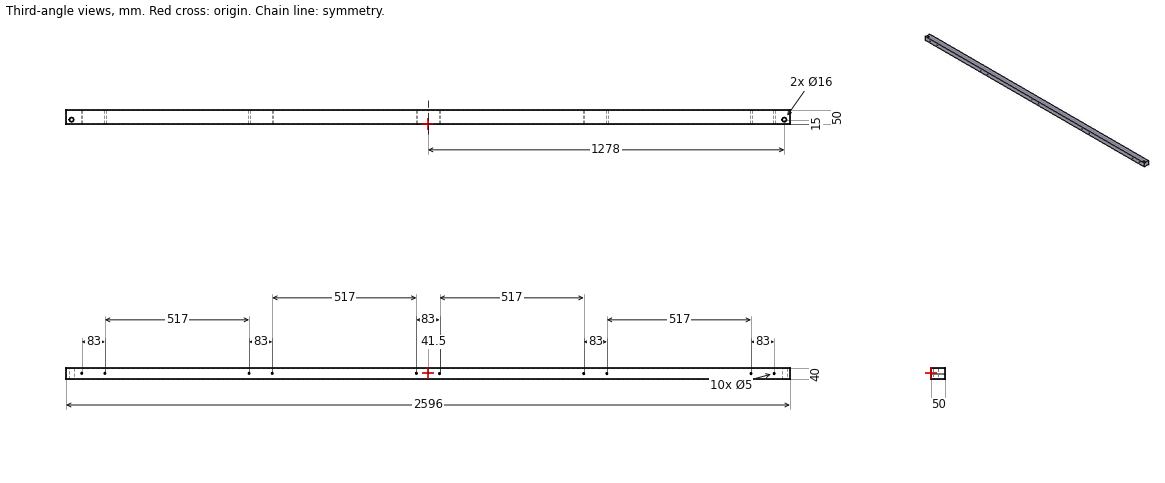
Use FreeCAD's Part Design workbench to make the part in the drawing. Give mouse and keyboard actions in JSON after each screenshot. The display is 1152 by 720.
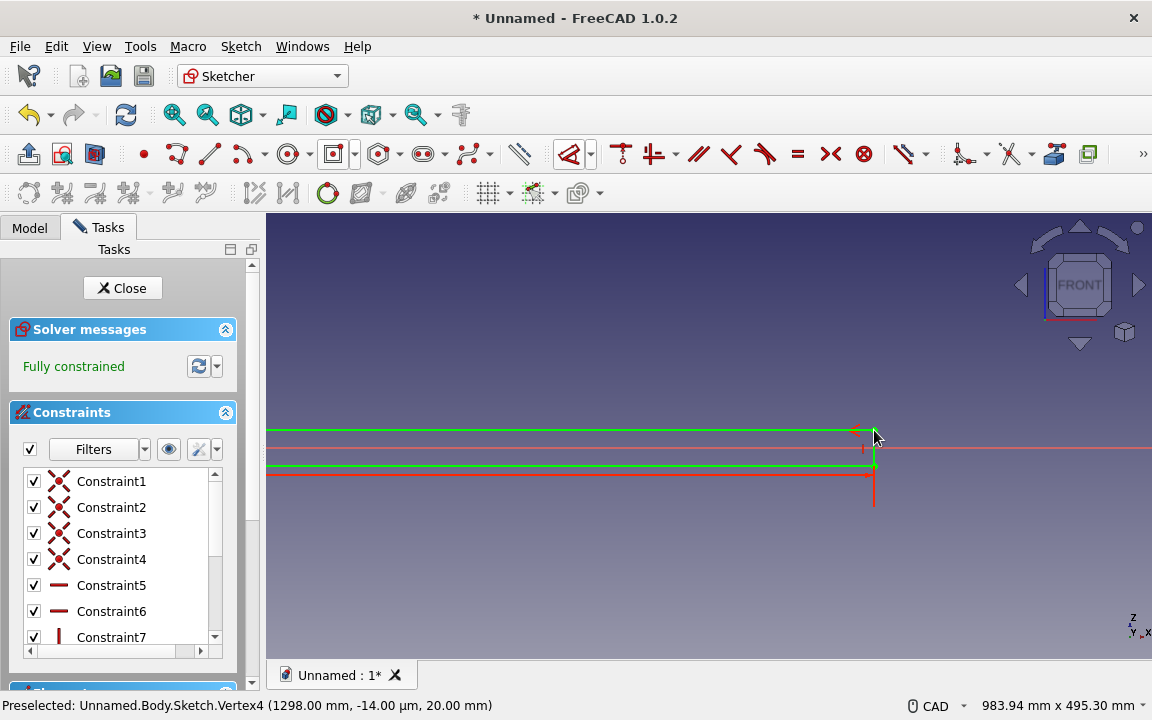
{"action": "left_click", "coordinate": [123, 288]}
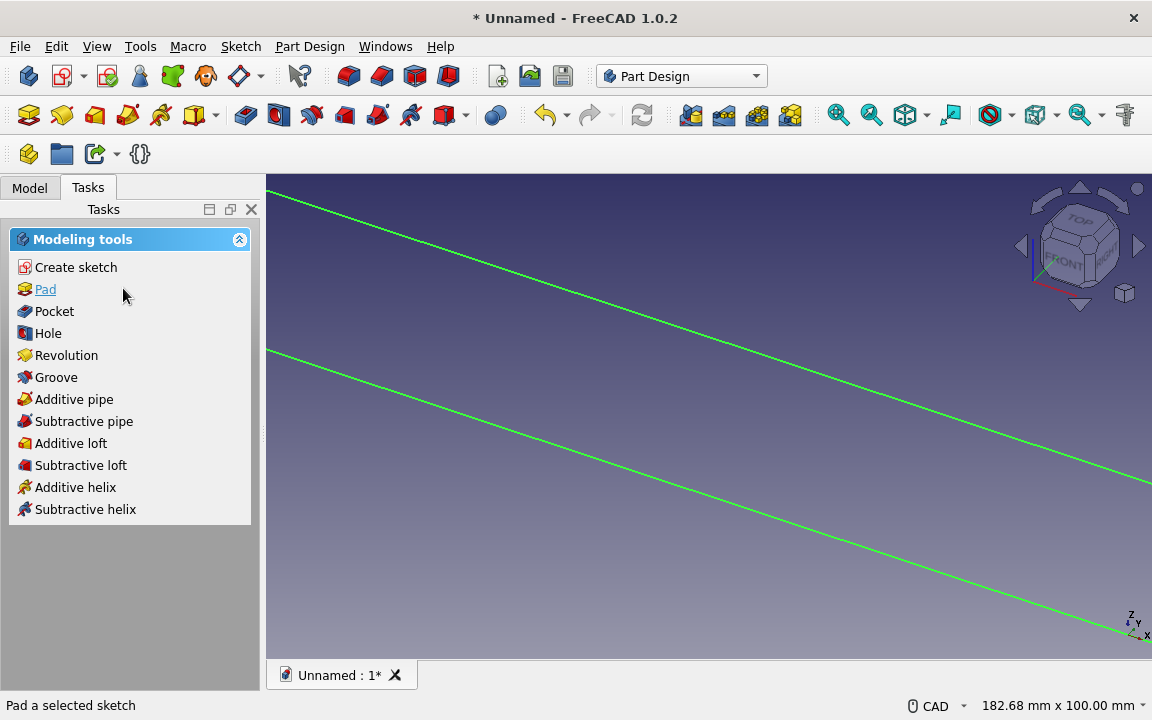
{"action": "left_click", "coordinate": [29, 116]}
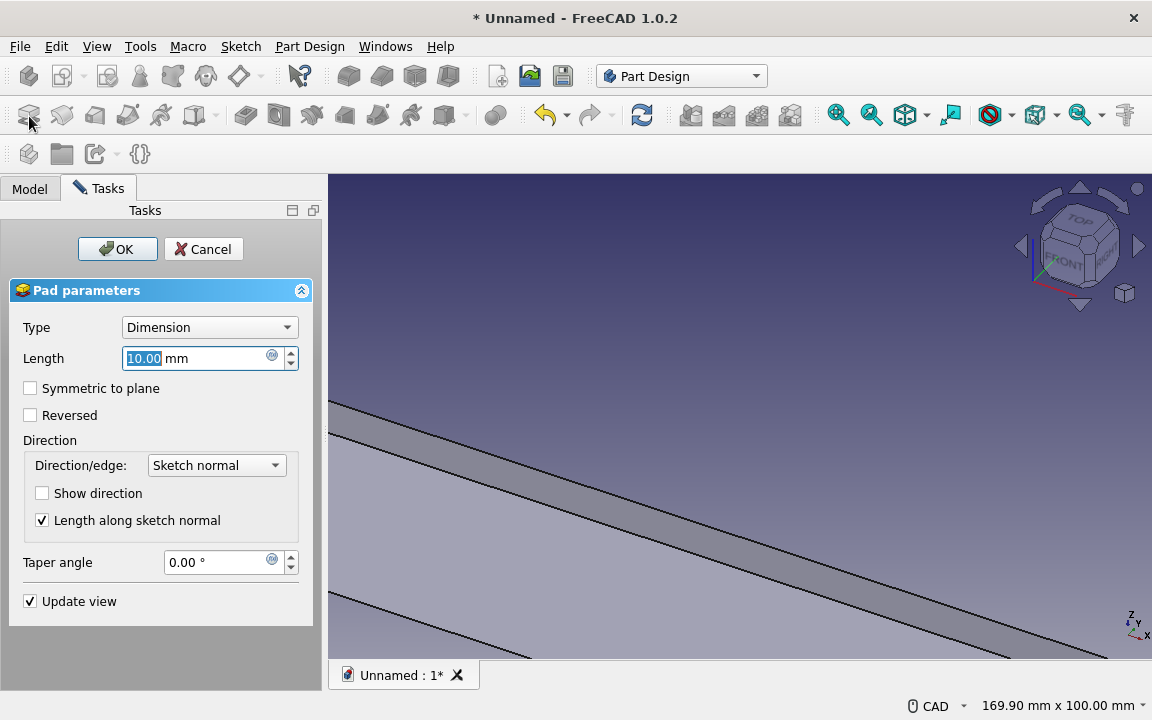
{"action": "type", "text": "50"}
{"action": "key", "text": "Tab"}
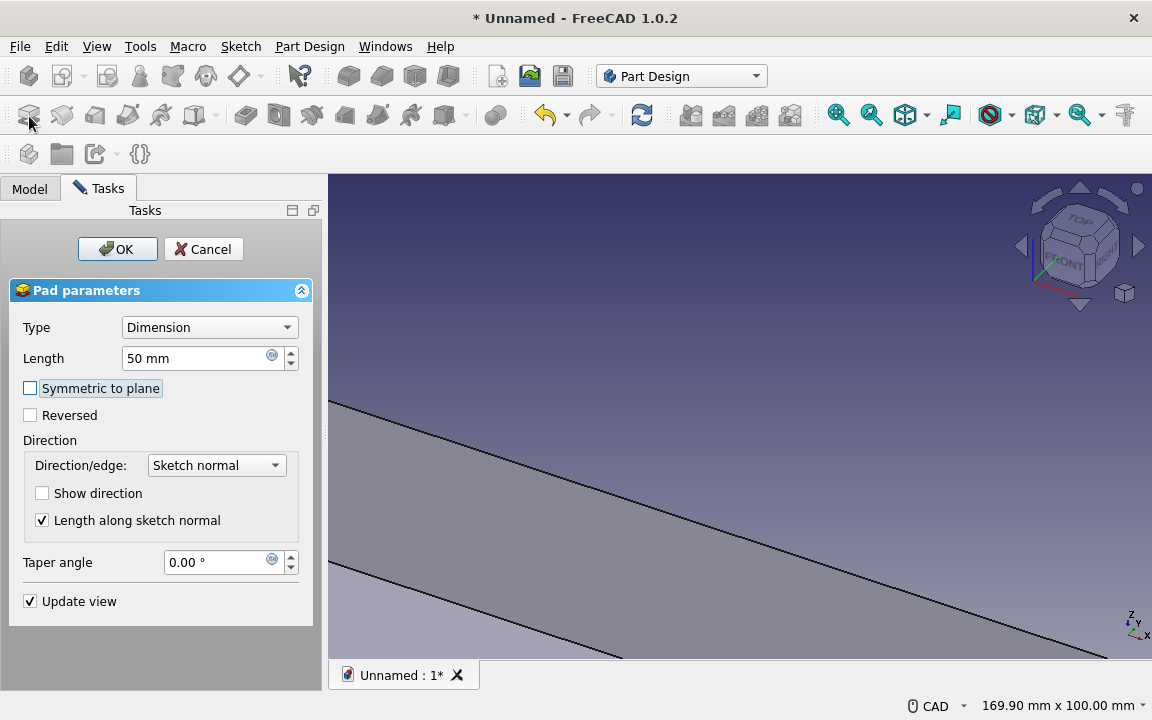
{"action": "left_click", "coordinate": [31, 415]}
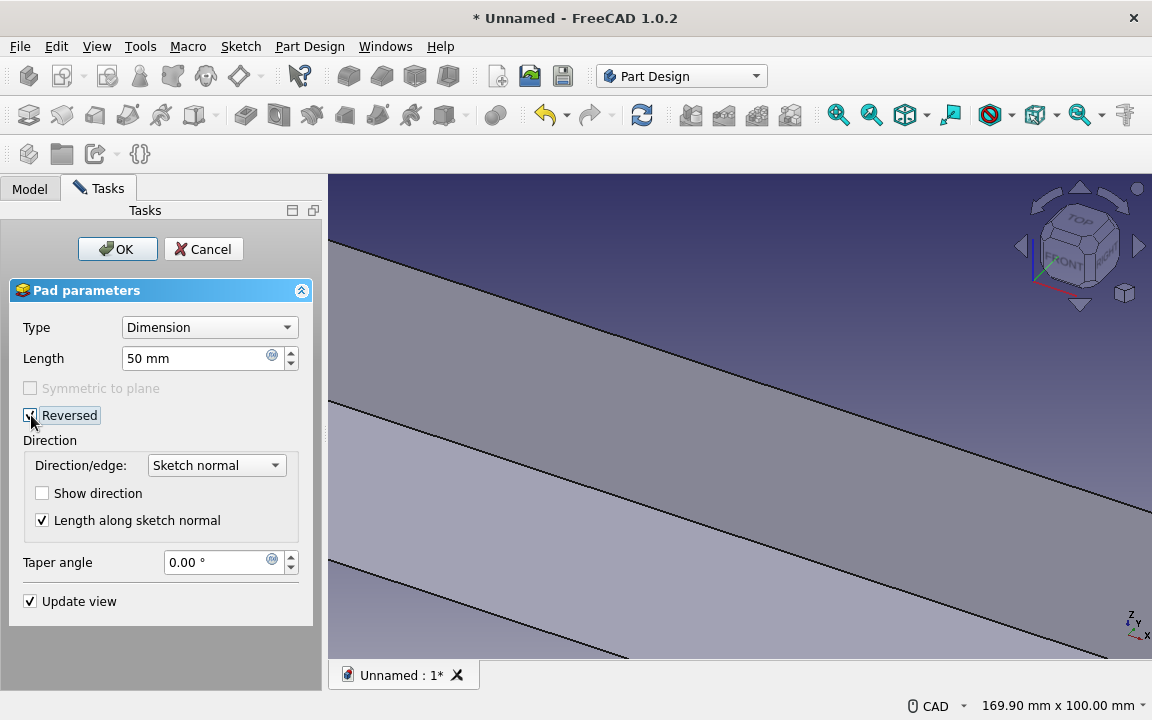
{"action": "left_click", "coordinate": [118, 249]}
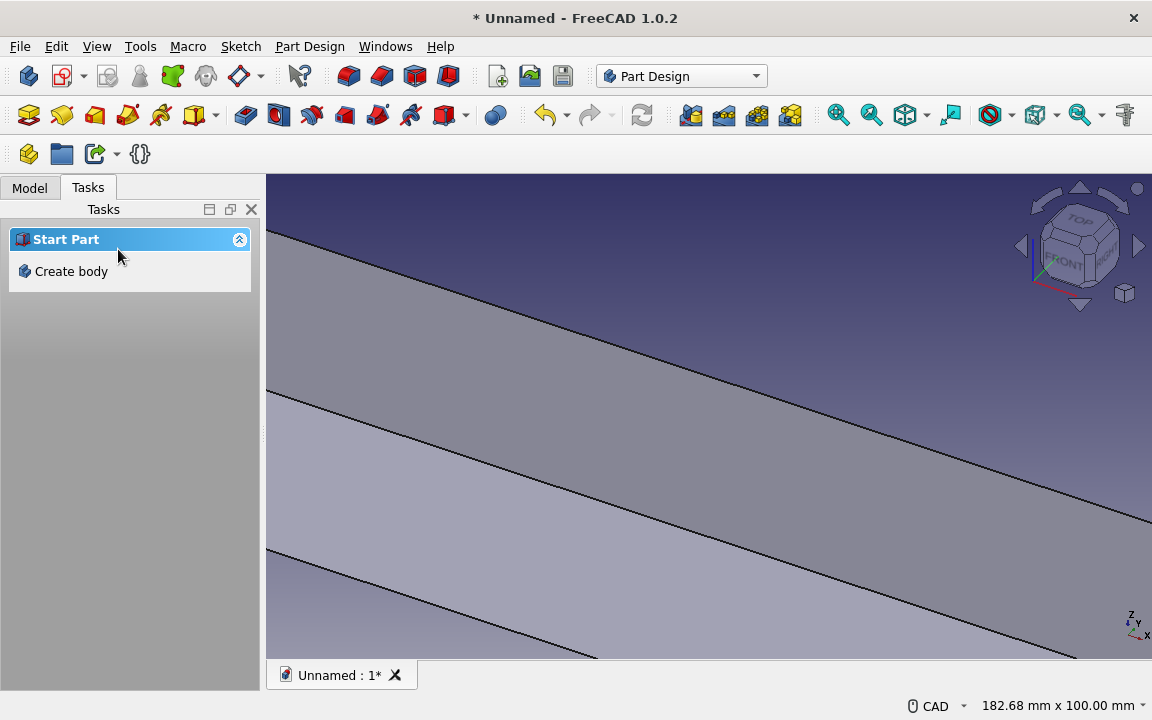
{"action": "left_click", "coordinate": [839, 116]}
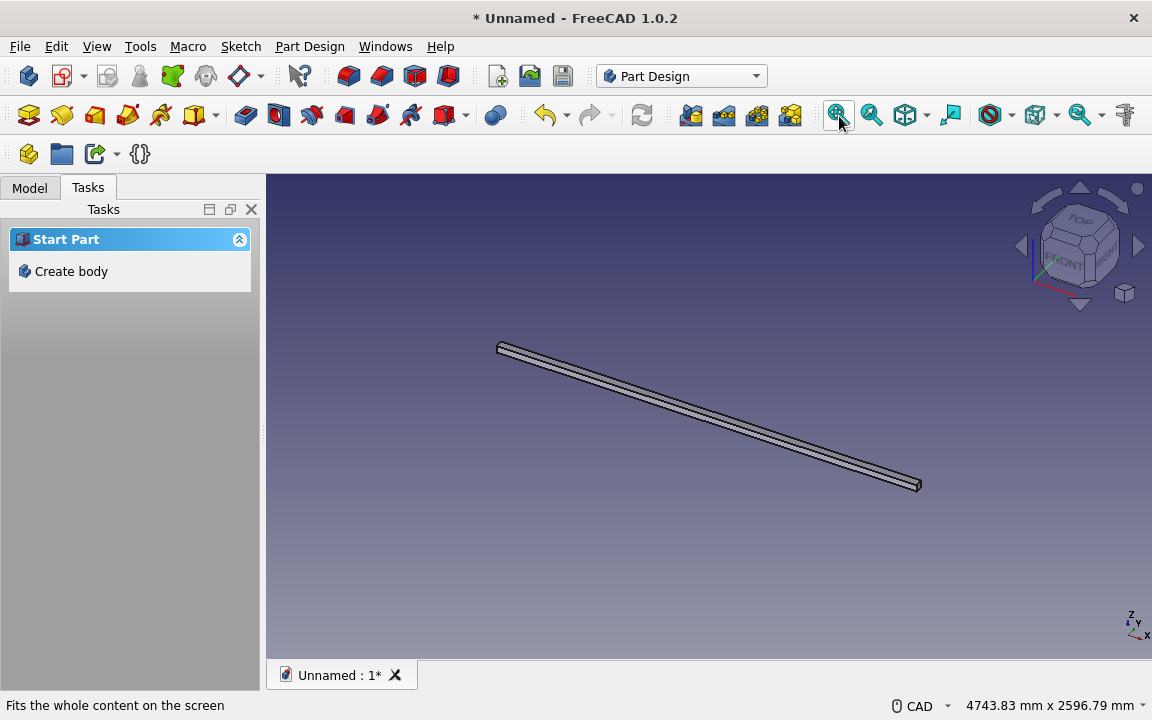
{"action": "scroll", "coordinate": [887, 477], "scroll_direction": "up", "scroll_amount": 6}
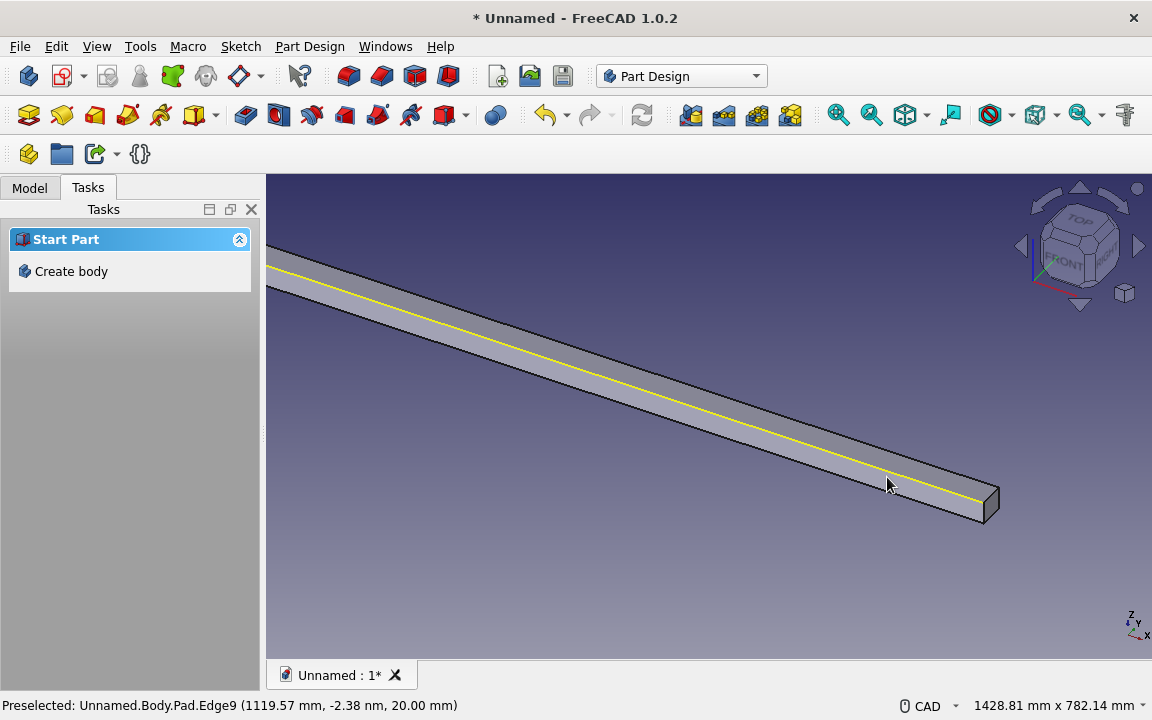
{"action": "left_click", "coordinate": [884, 479]}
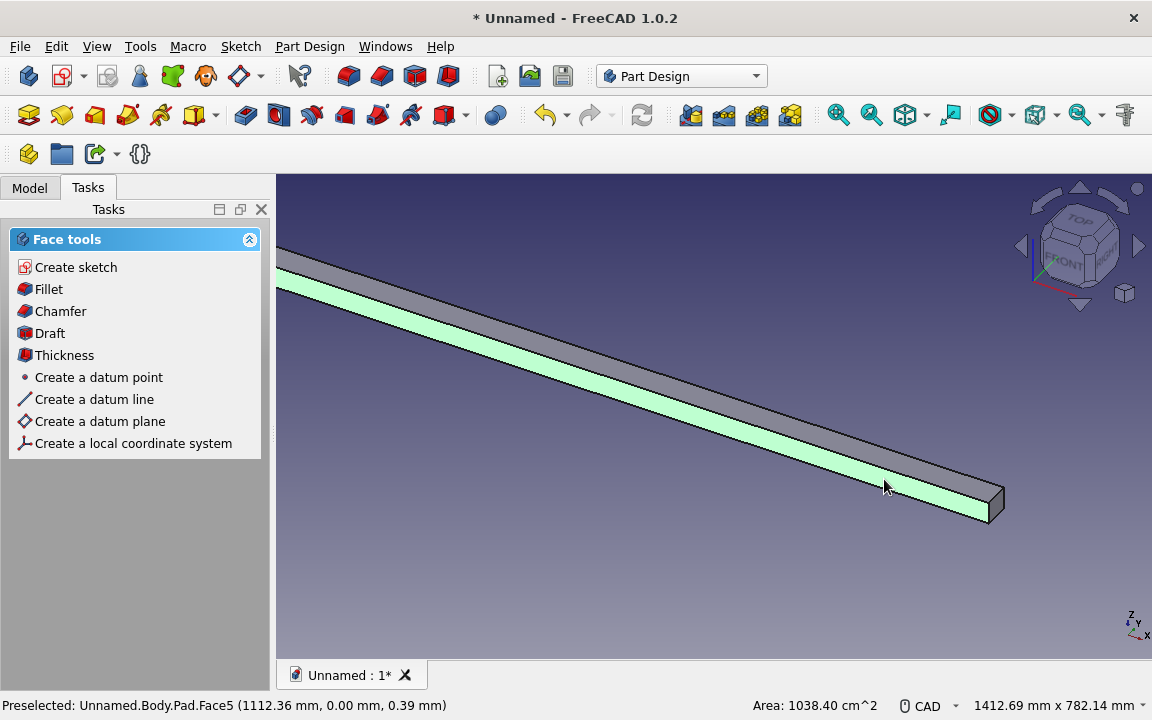
{"action": "left_click", "coordinate": [62, 76]}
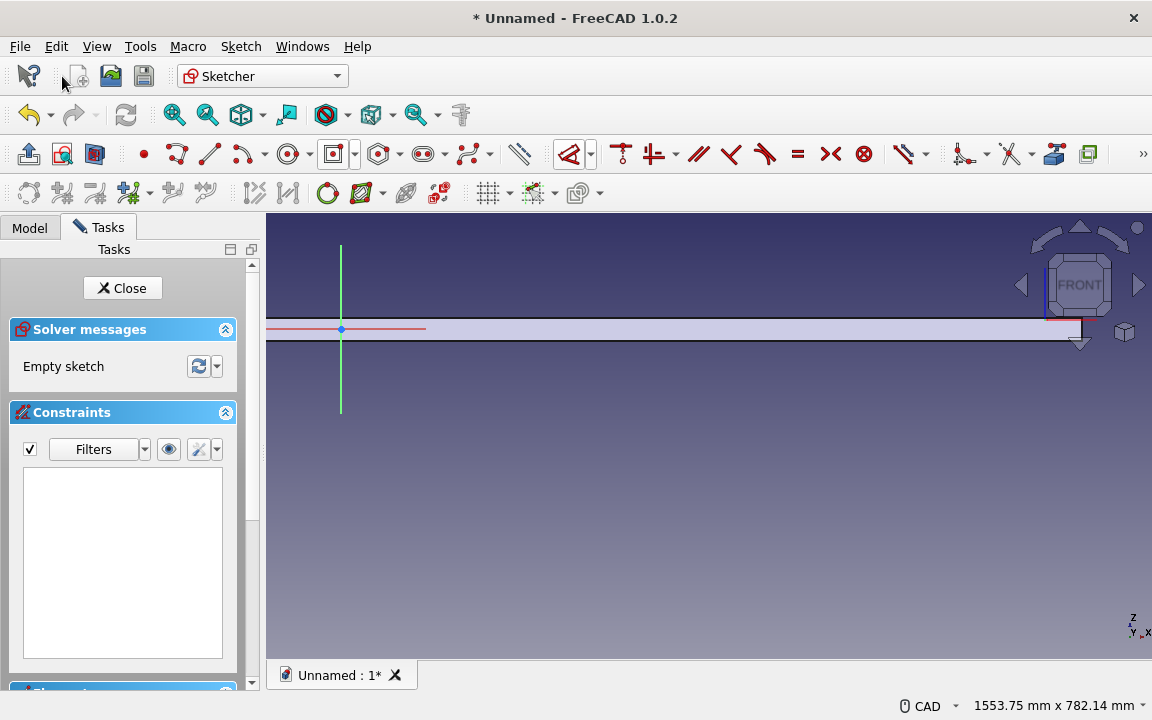
{"action": "scroll", "coordinate": [815, 498], "scroll_direction": "down", "scroll_amount": 5}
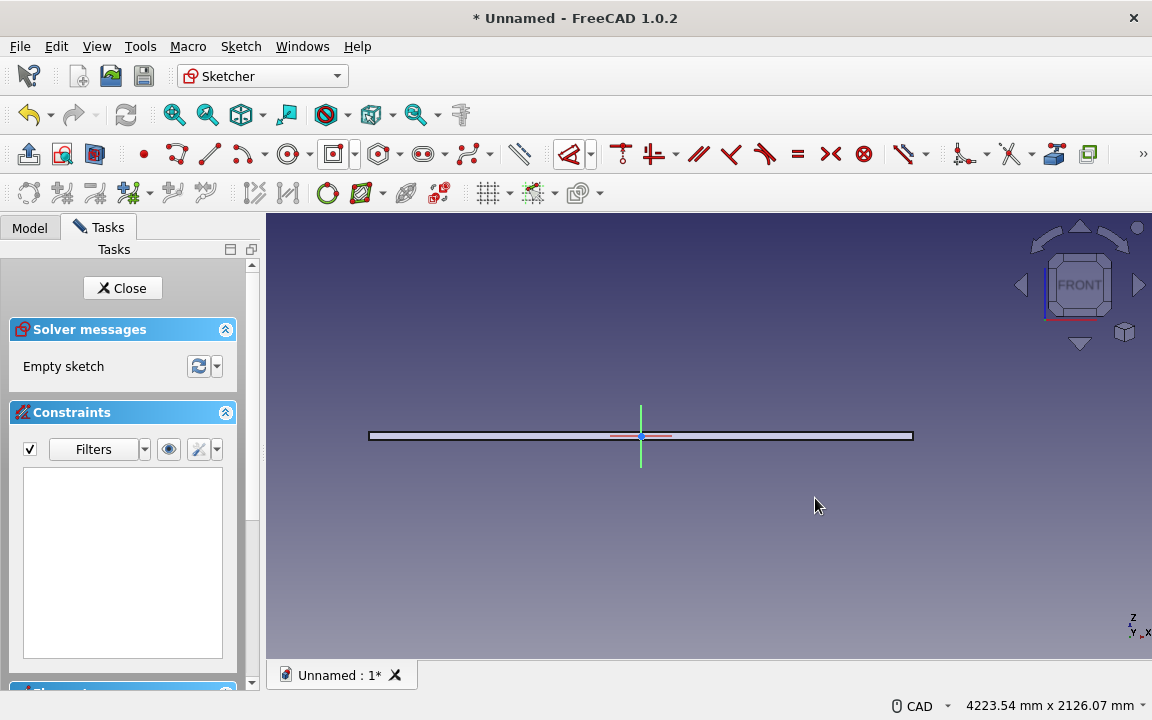
{"action": "left_click", "coordinate": [288, 154]}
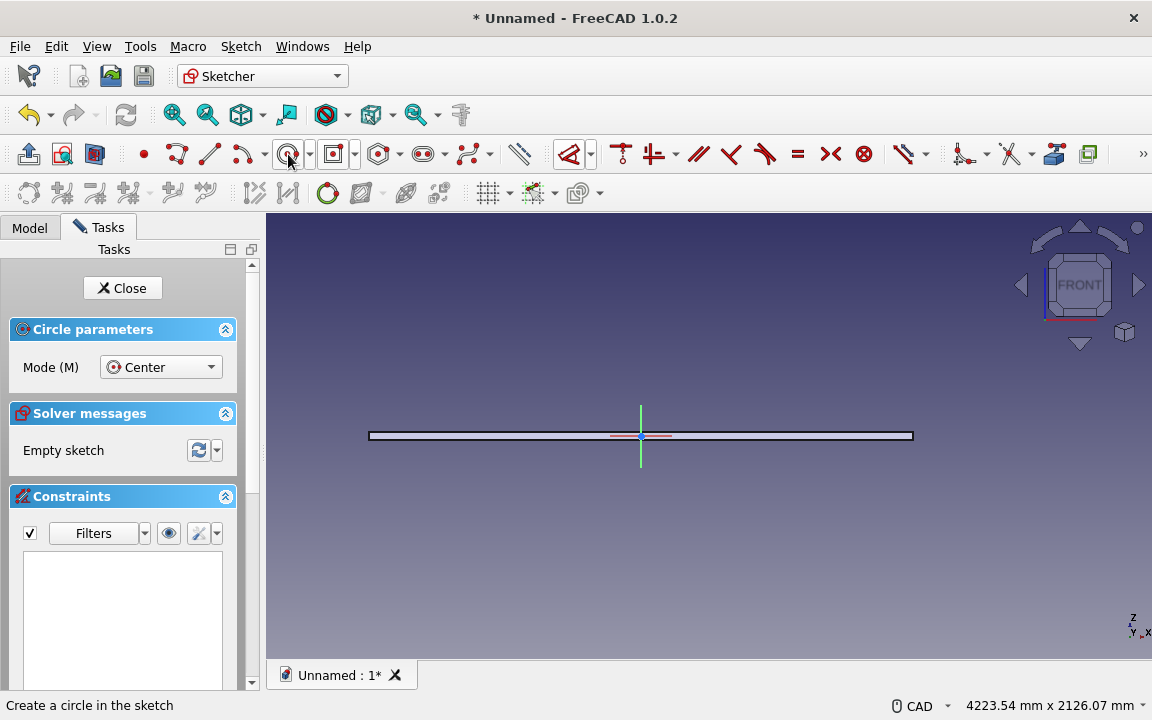
{"action": "scroll", "coordinate": [902, 436], "scroll_direction": "up", "scroll_amount": 19}